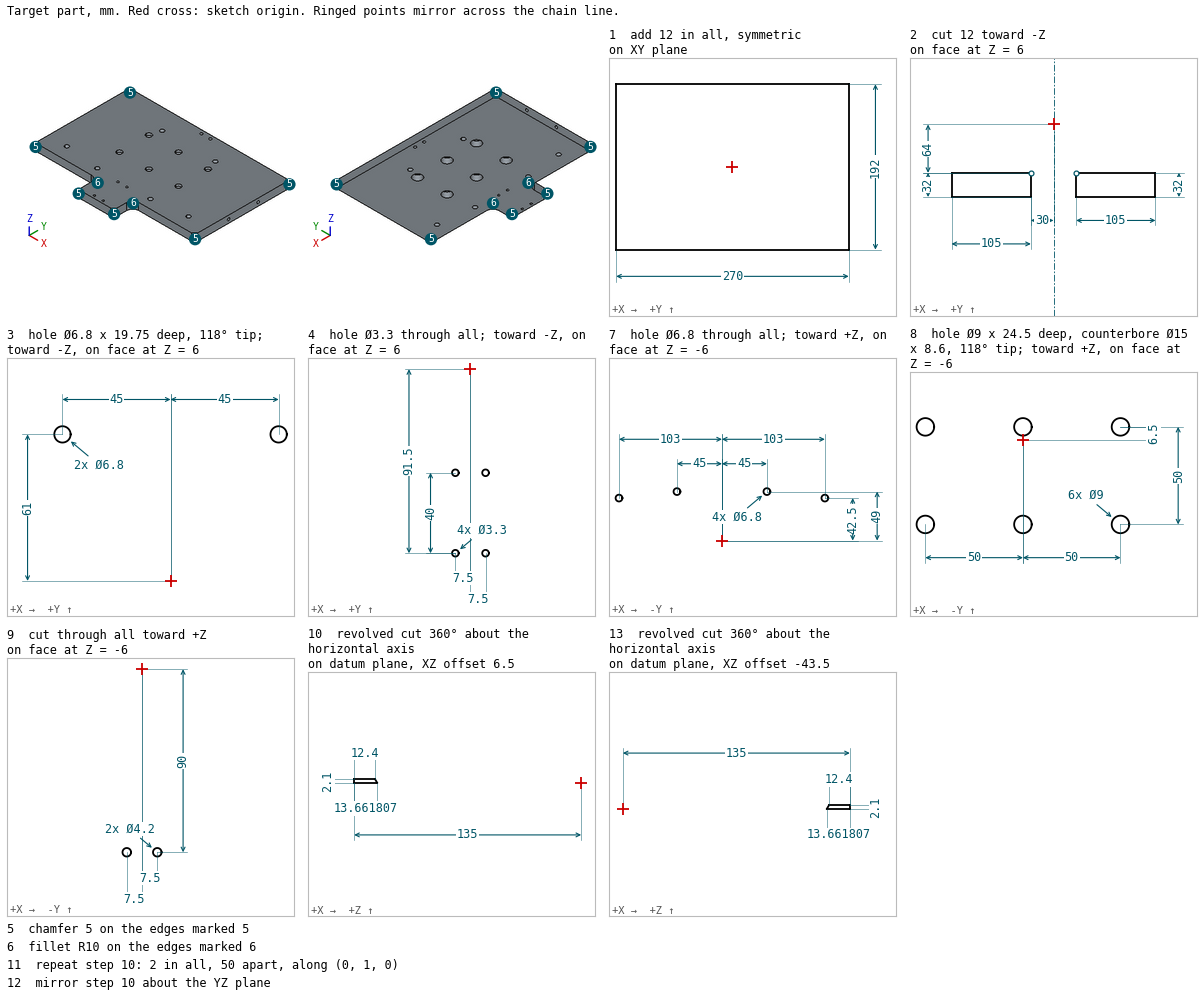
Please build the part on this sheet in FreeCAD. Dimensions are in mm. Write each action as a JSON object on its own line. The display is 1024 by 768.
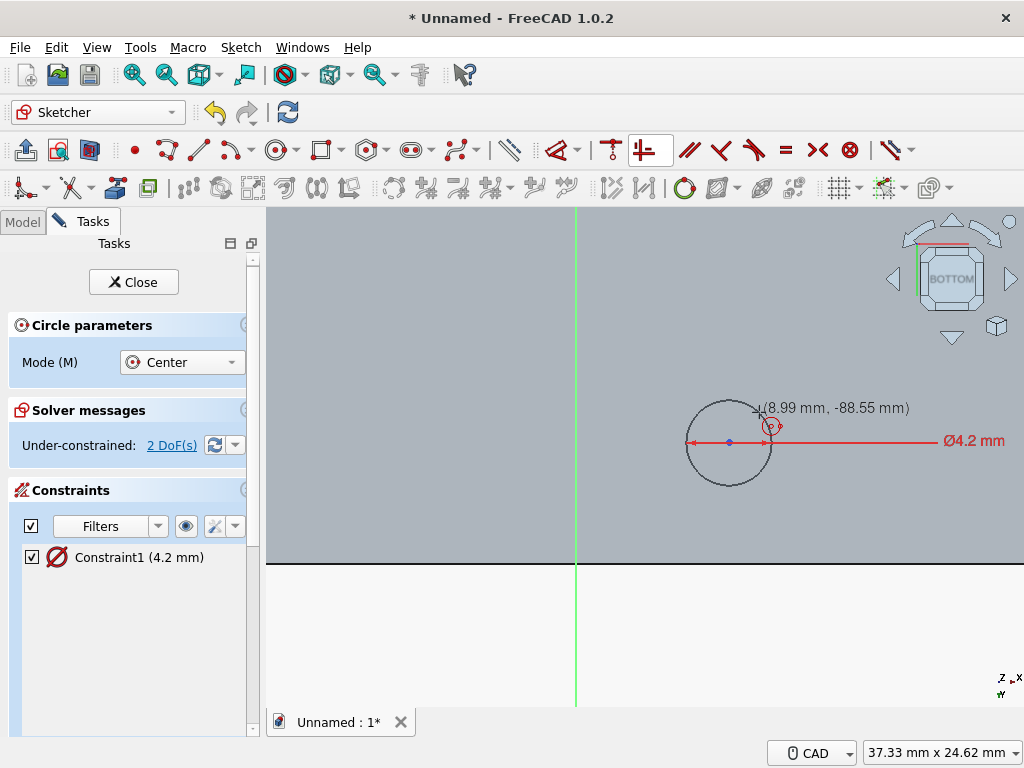
{"action": "left_click", "coordinate": [424, 442]}
{"action": "mouse_move", "coordinate": [454, 412]}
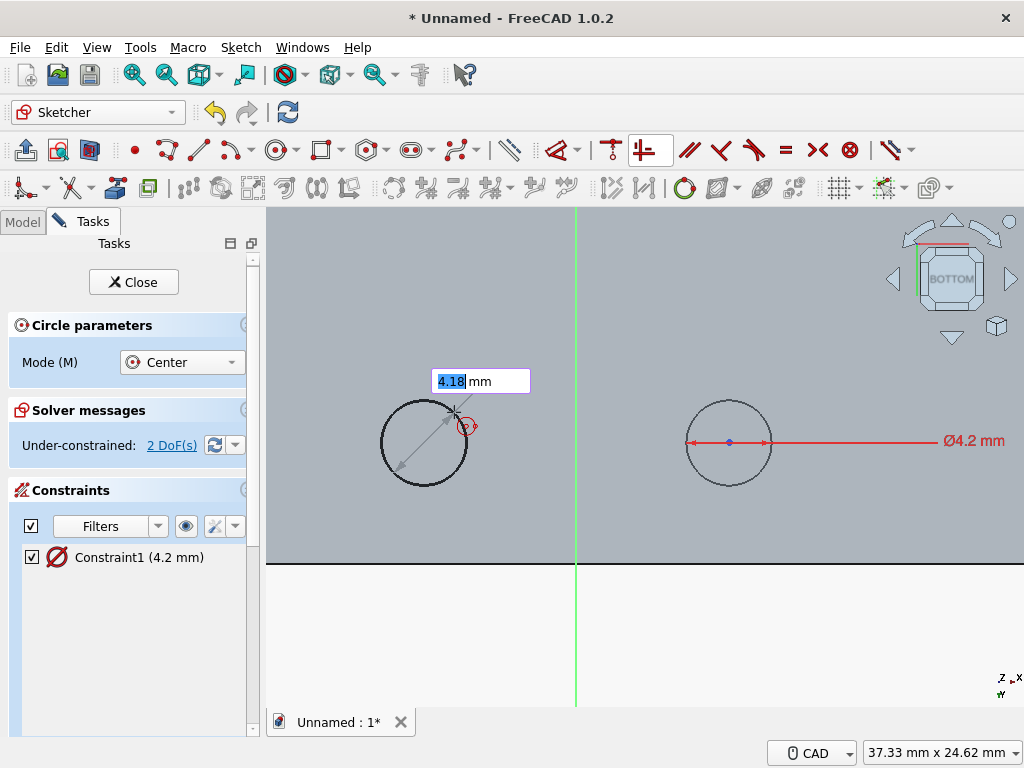
{"action": "type", "text": "4.2"}
{"action": "key", "text": "Return"}
{"action": "key", "text": "Escape"}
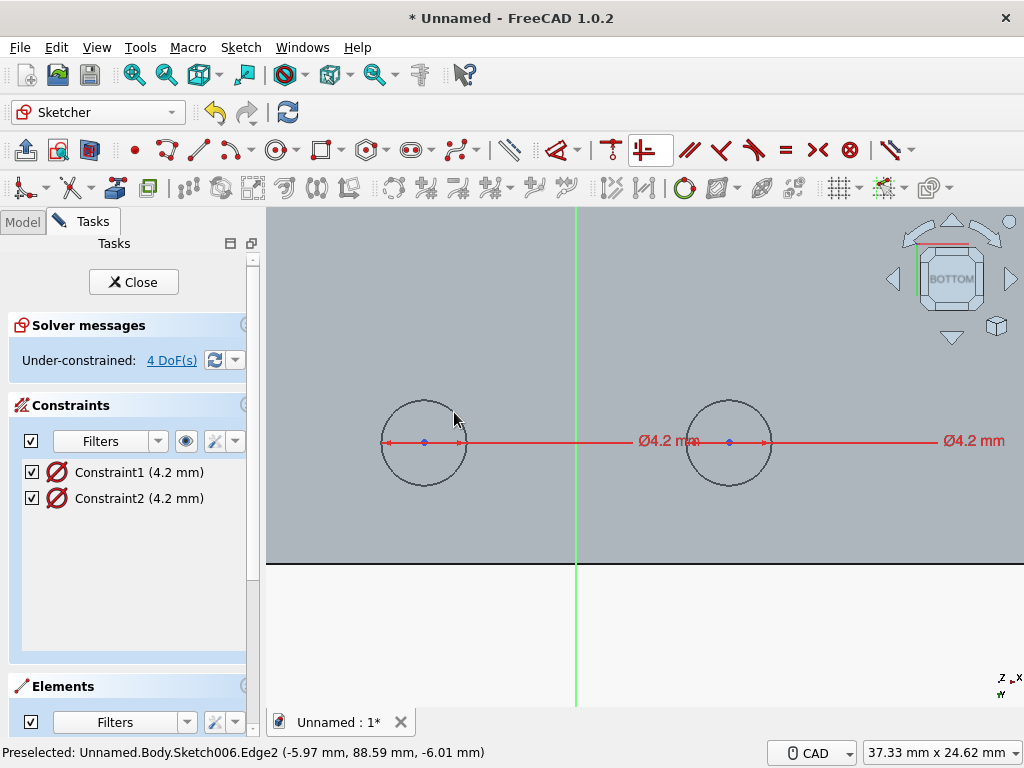
{"action": "left_click", "coordinate": [729, 443]}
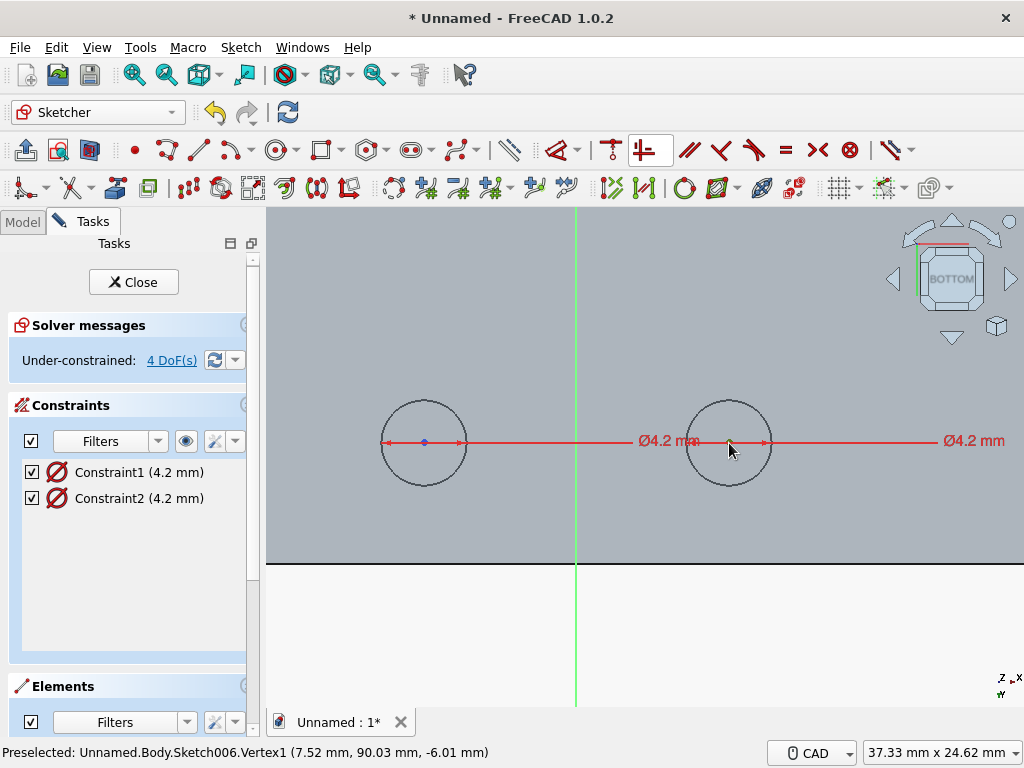
{"action": "left_click", "coordinate": [424, 443]}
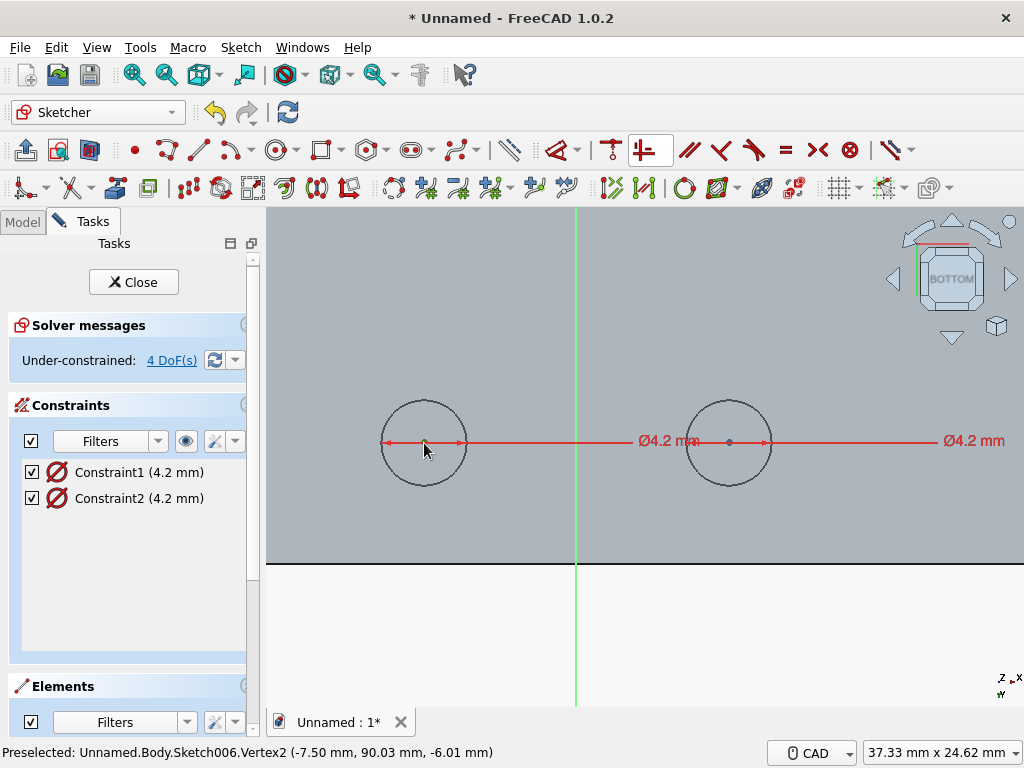
{"action": "key", "text": "h"}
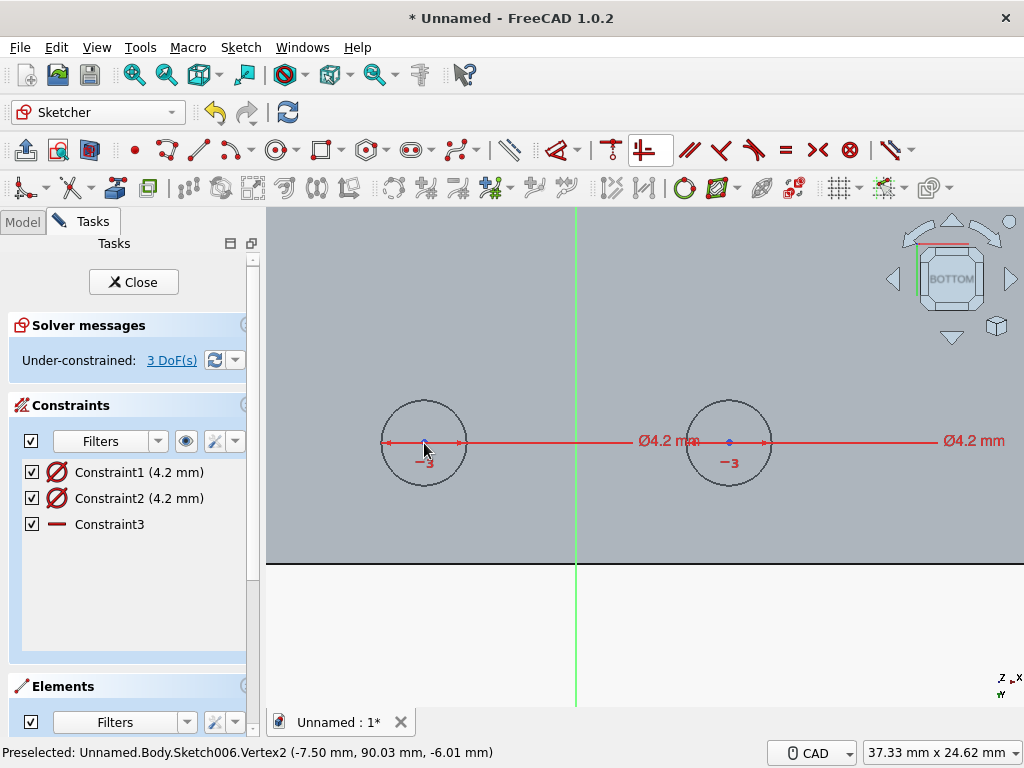
{"action": "key", "text": "d"}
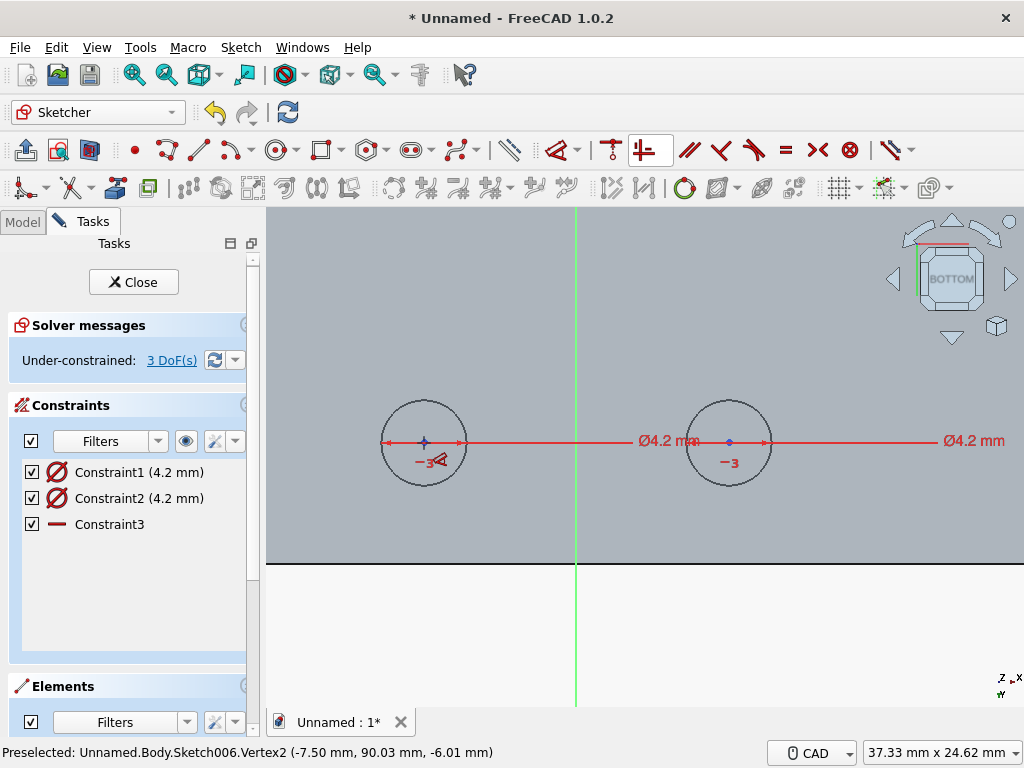
{"action": "left_click", "coordinate": [729, 443]}
{"action": "left_click", "coordinate": [763, 339]}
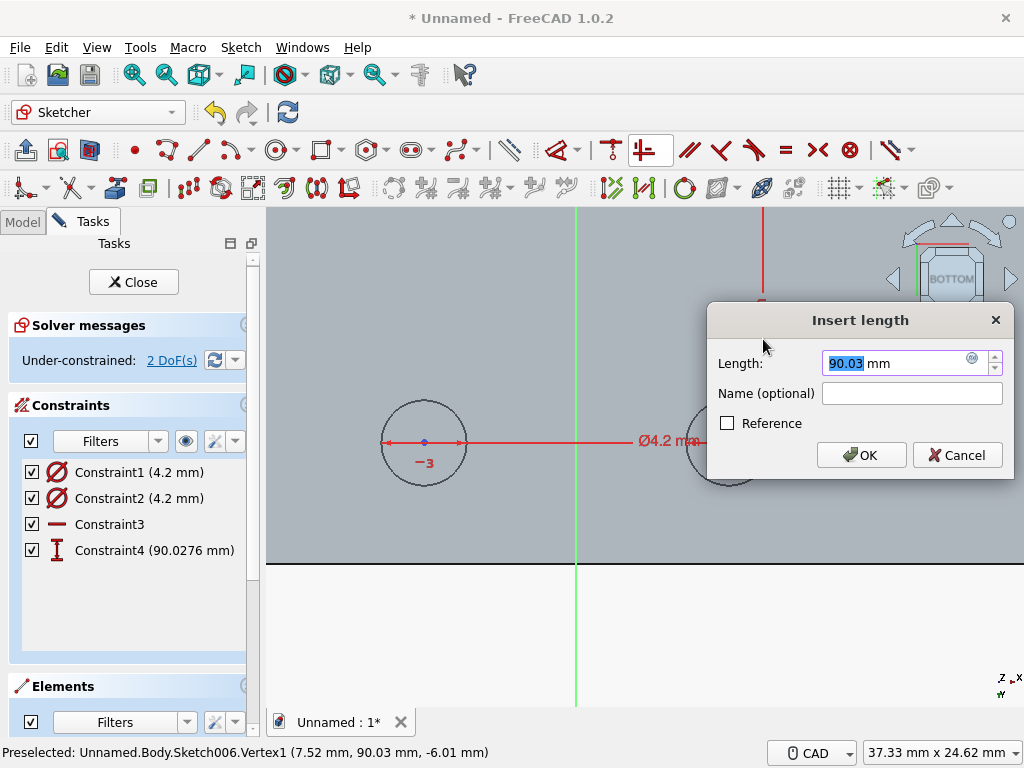
{"action": "type", "text": "90"}
{"action": "key", "text": "Return"}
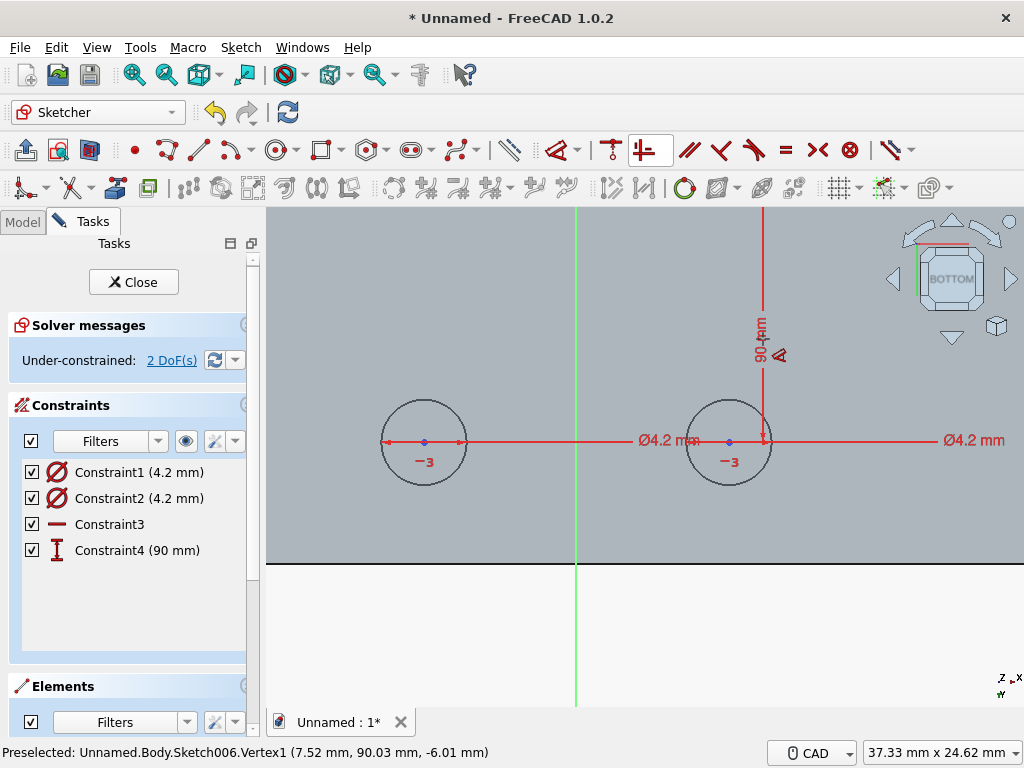
{"action": "left_click", "coordinate": [729, 442]}
{"action": "left_click", "coordinate": [653, 476]}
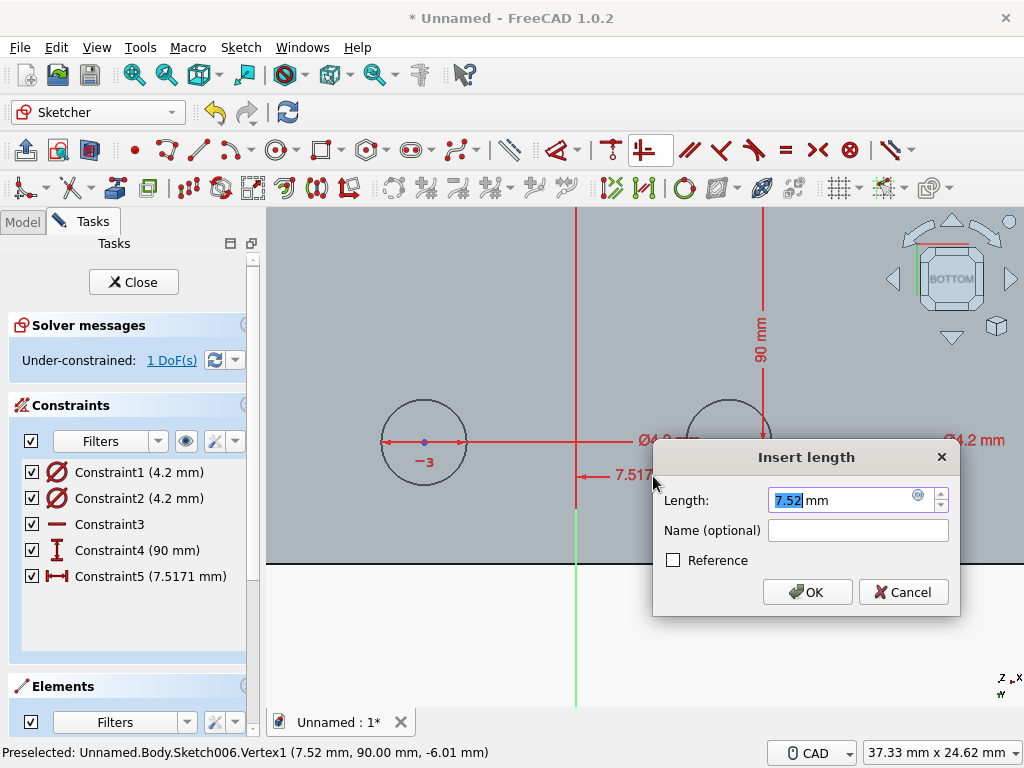
{"action": "type", "text": "7.5"}
{"action": "key", "text": "Return"}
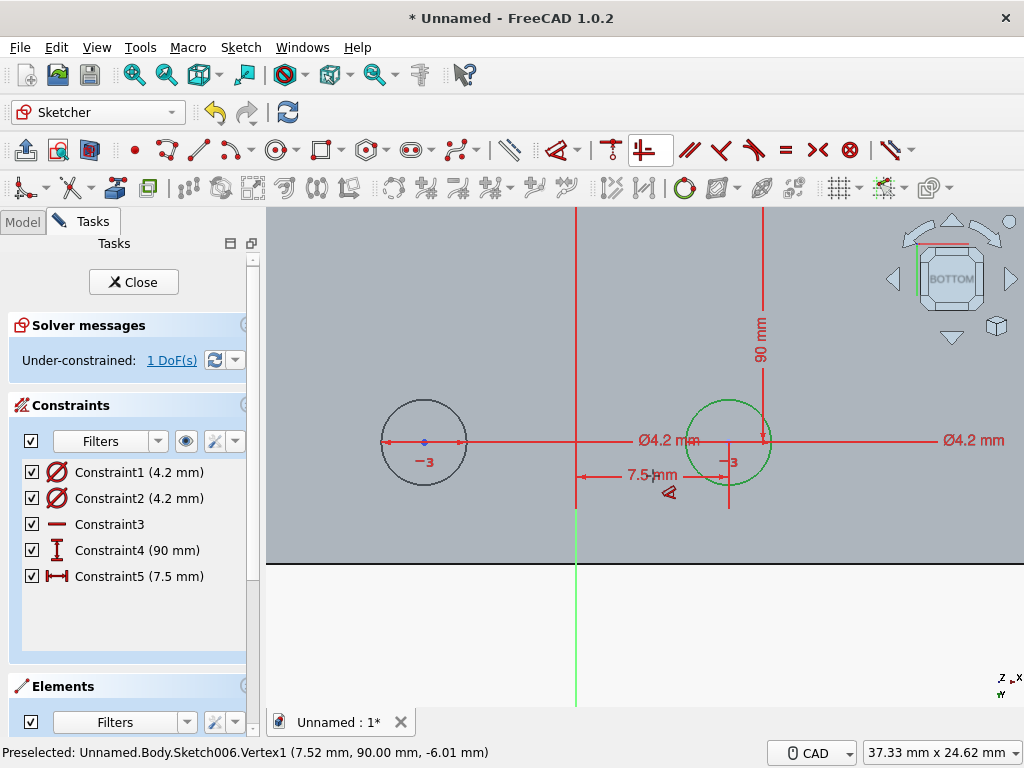
{"action": "left_click", "coordinate": [424, 442]}
{"action": "left_click", "coordinate": [500, 476]}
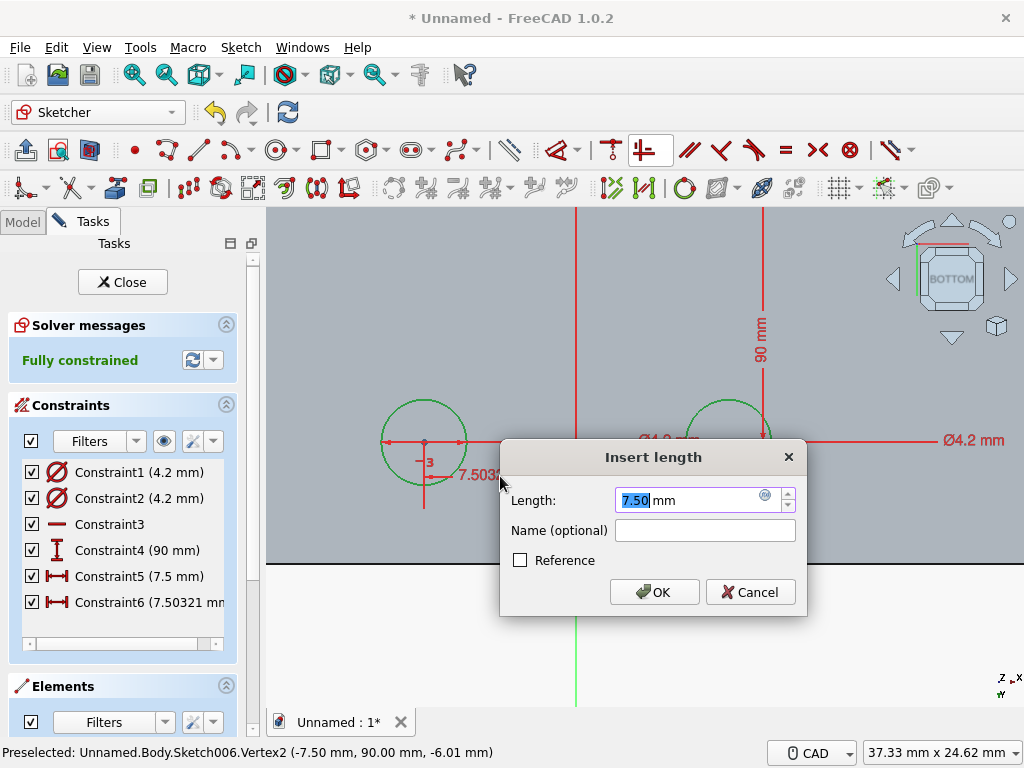
{"action": "type", "text": "7.5"}
{"action": "key", "text": "Return"}
{"action": "key", "text": "Escape"}